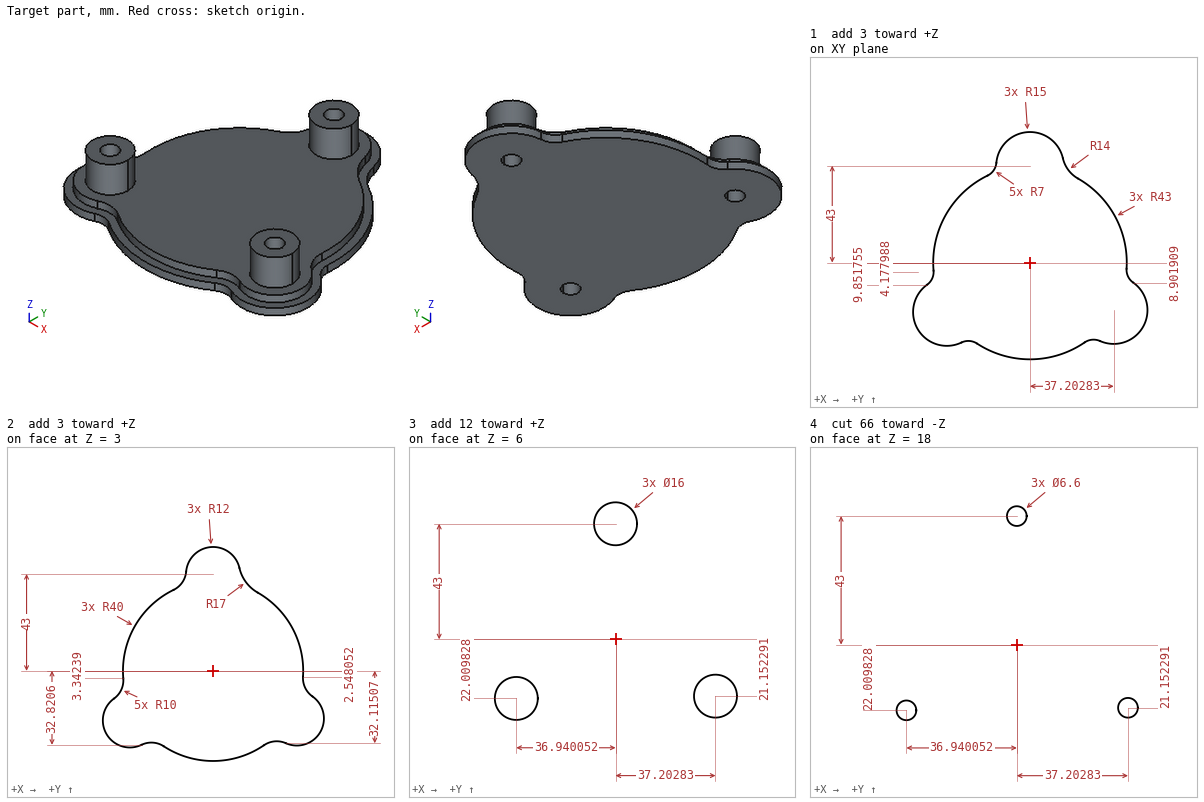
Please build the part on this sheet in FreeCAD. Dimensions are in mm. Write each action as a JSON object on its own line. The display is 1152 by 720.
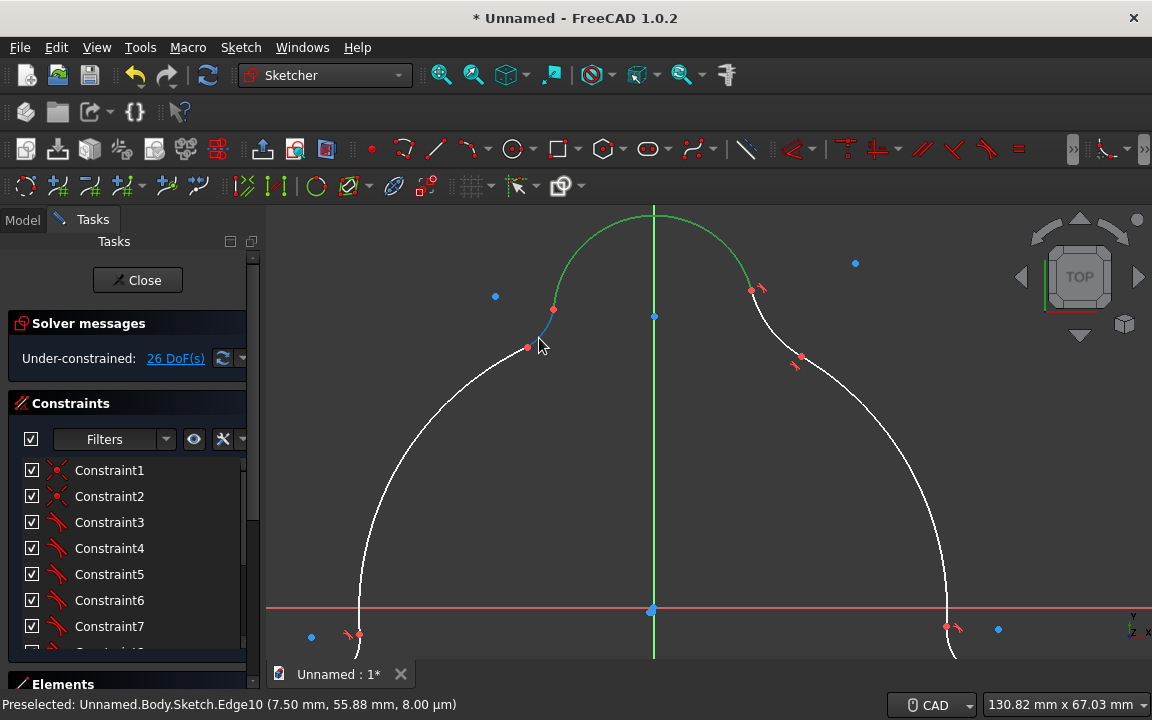
{"action": "left_click", "coordinate": [538, 338]}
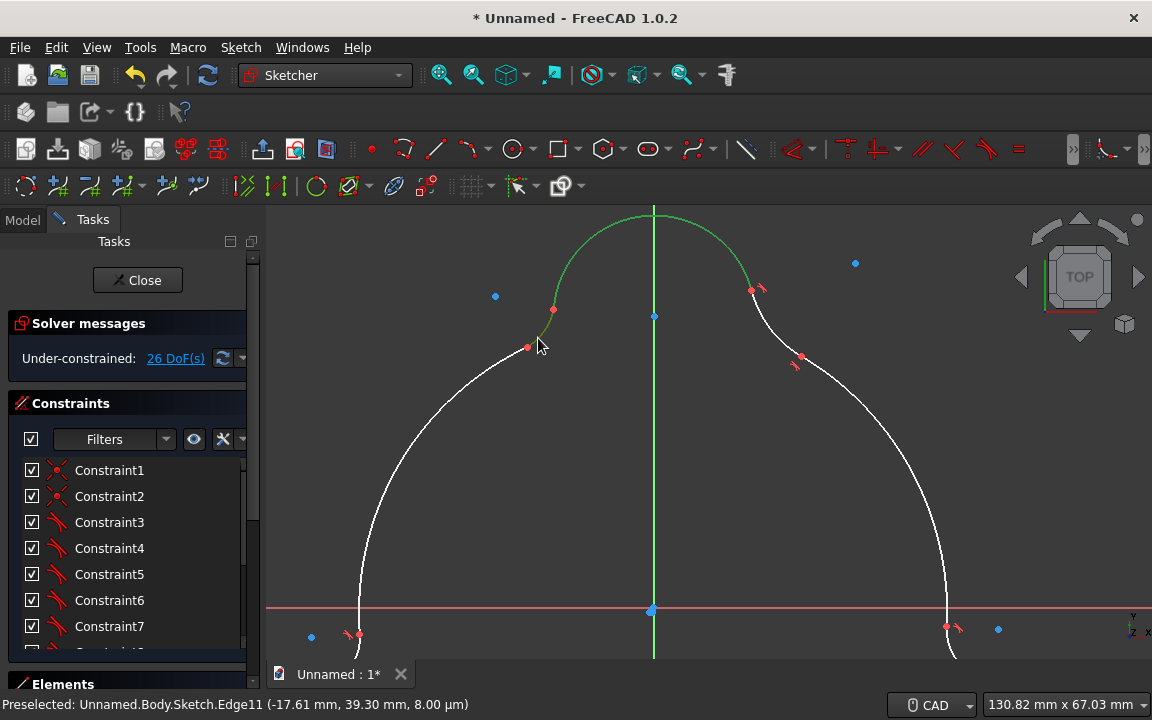
{"action": "left_click", "coordinate": [988, 150]}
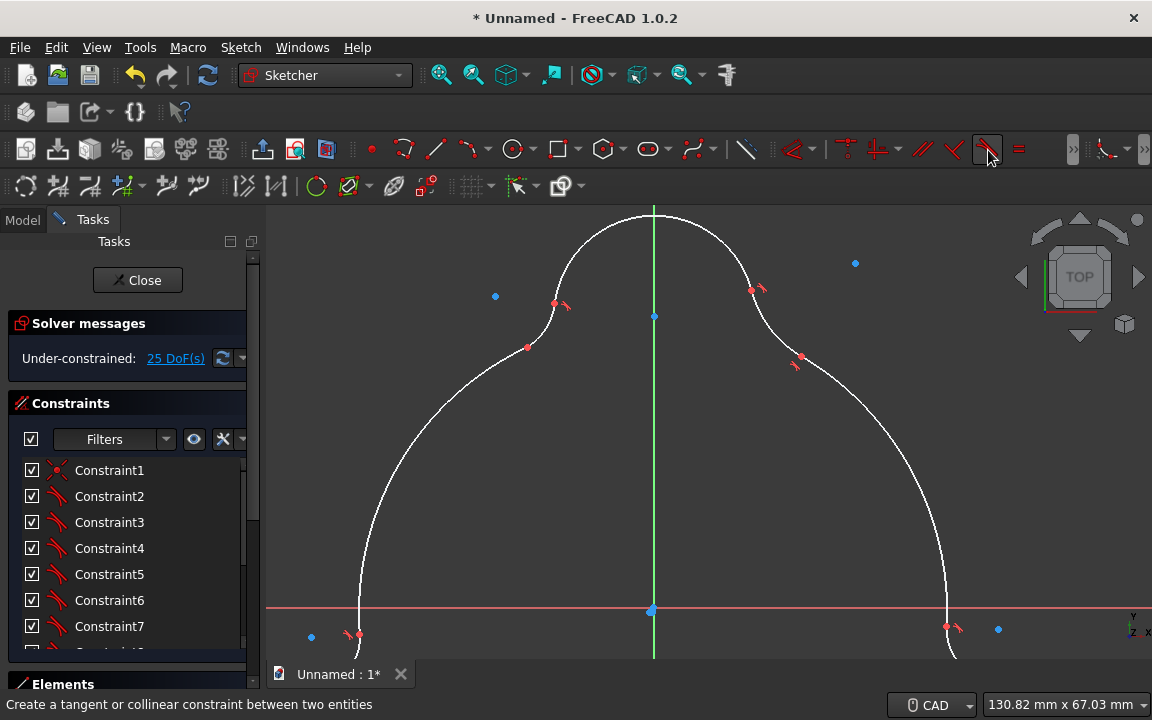
{"action": "left_click", "coordinate": [539, 337]}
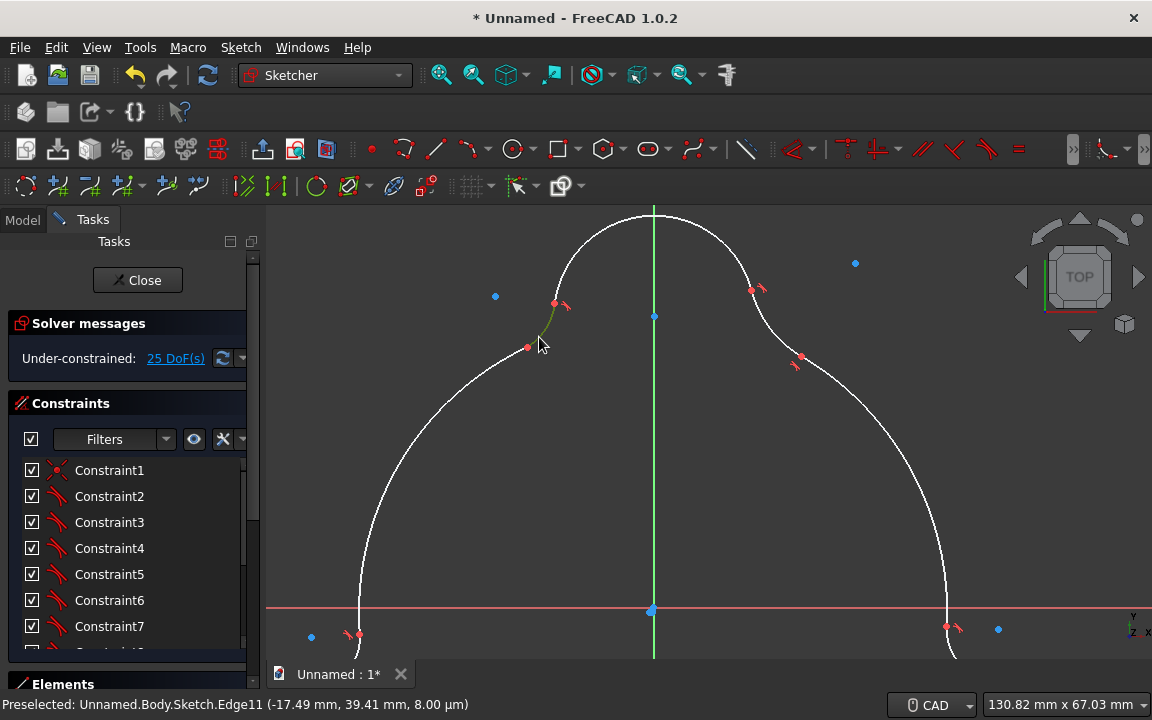
{"action": "left_click", "coordinate": [441, 408]}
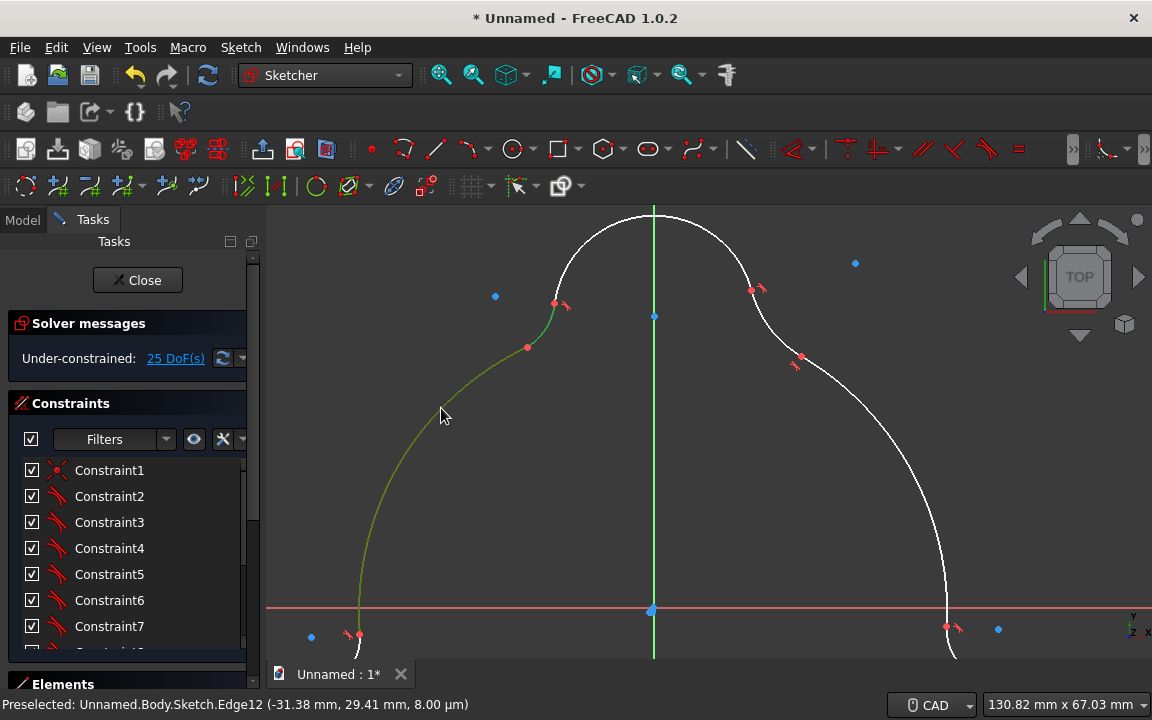
{"action": "left_click", "coordinate": [988, 150]}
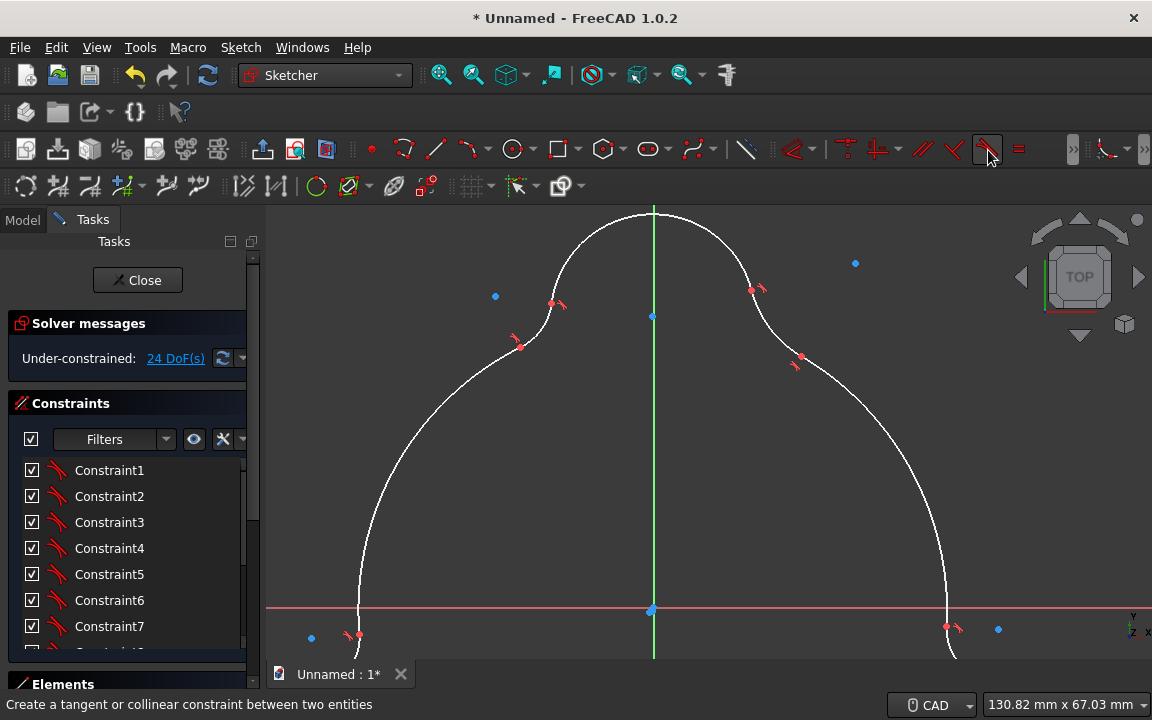
{"action": "scroll", "coordinate": [628, 330], "scroll_direction": "down", "scroll_amount": 4}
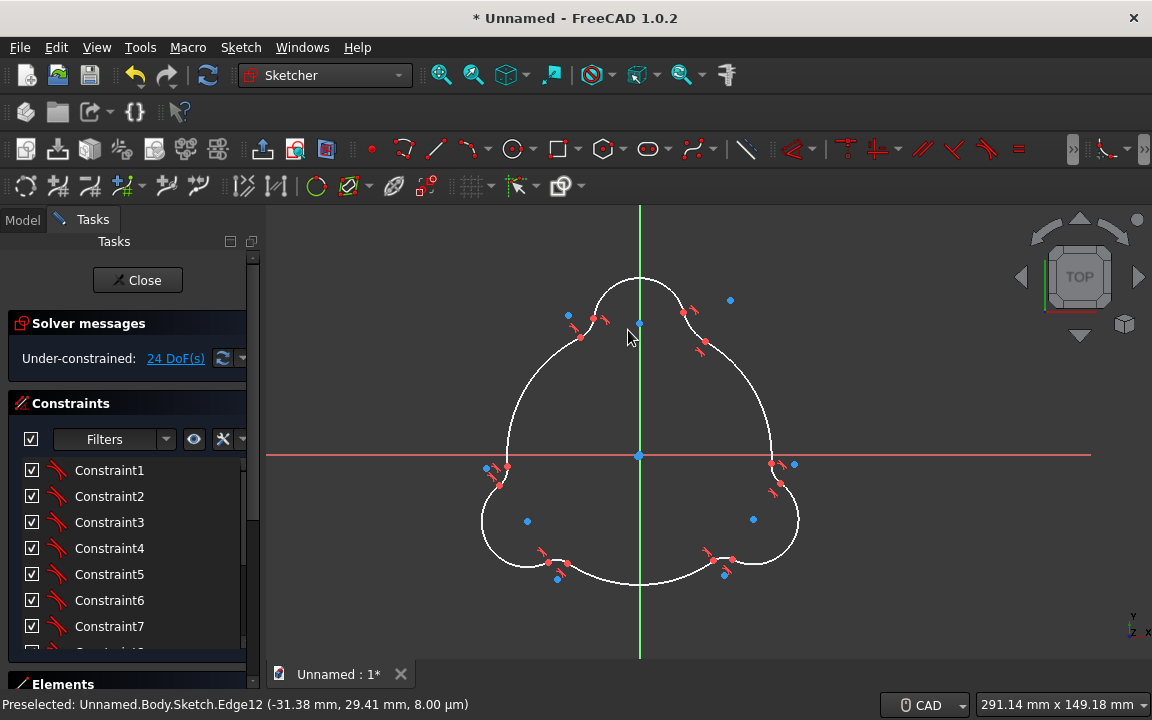
{"action": "left_click", "coordinate": [610, 582]}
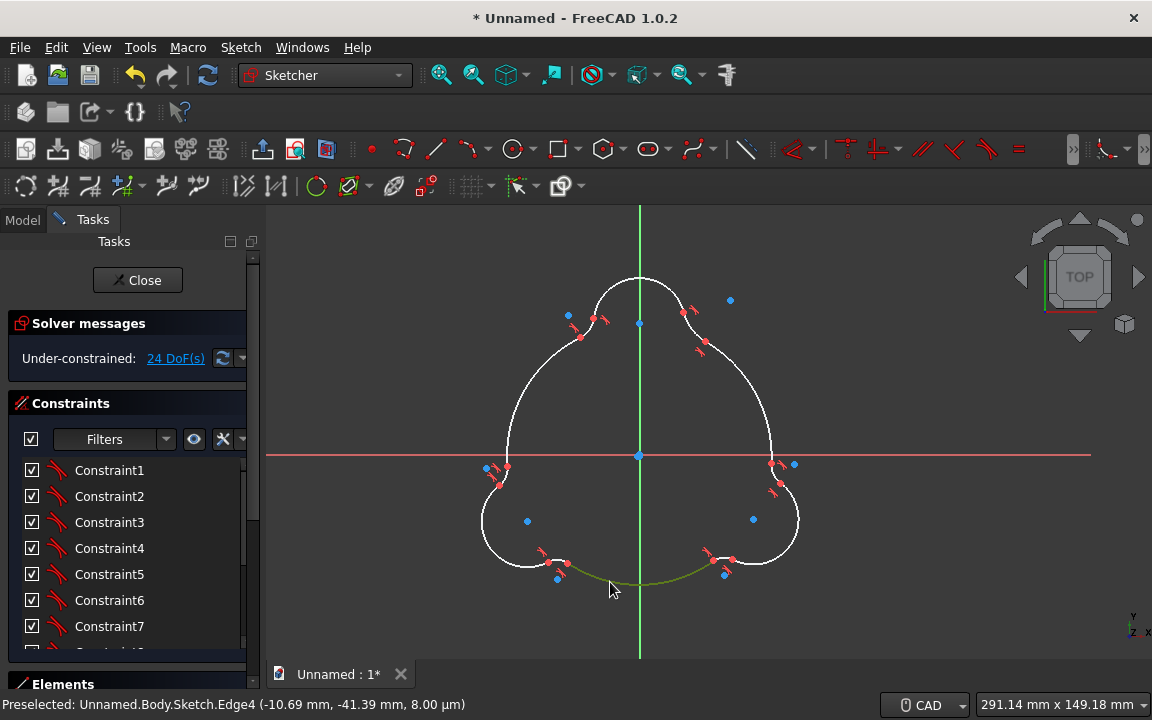
{"action": "left_click", "coordinate": [767, 420]}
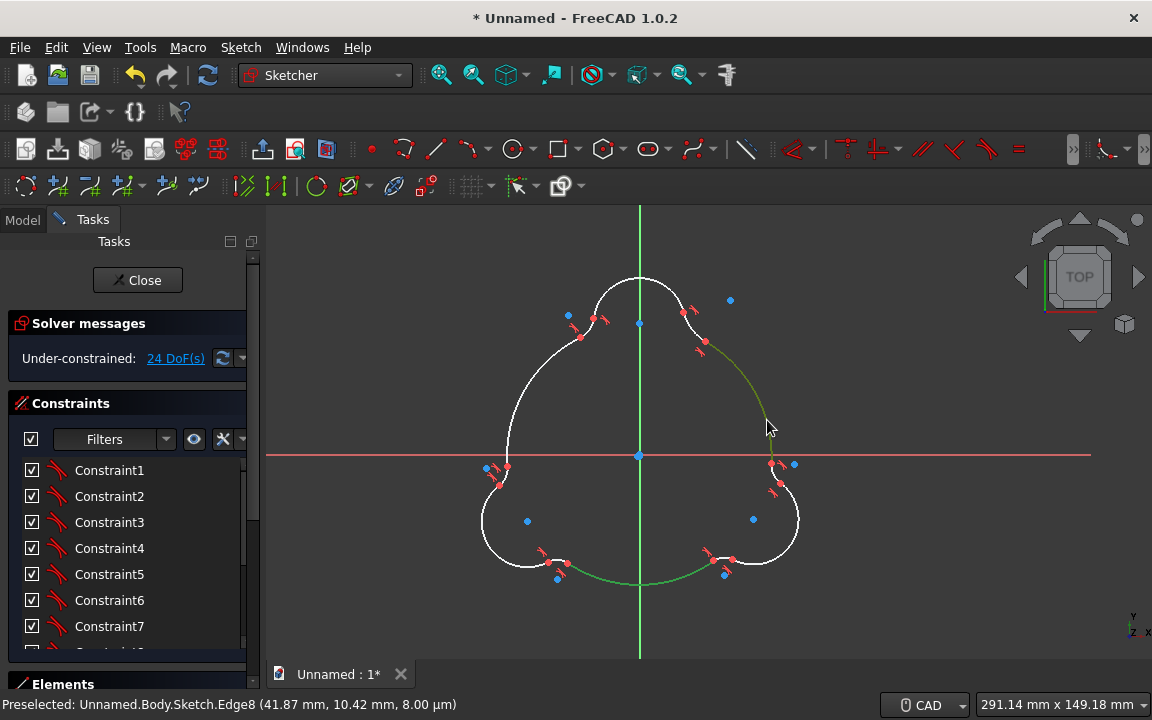
{"action": "left_click", "coordinate": [846, 150]}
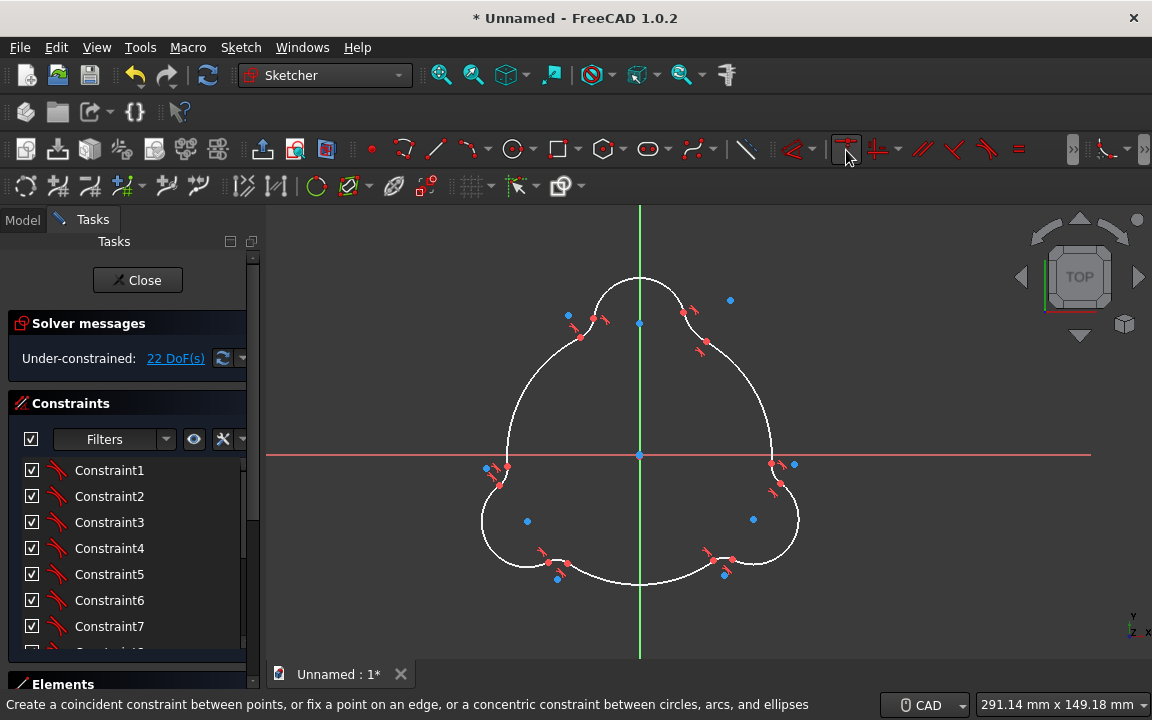
{"action": "left_click", "coordinate": [610, 582]}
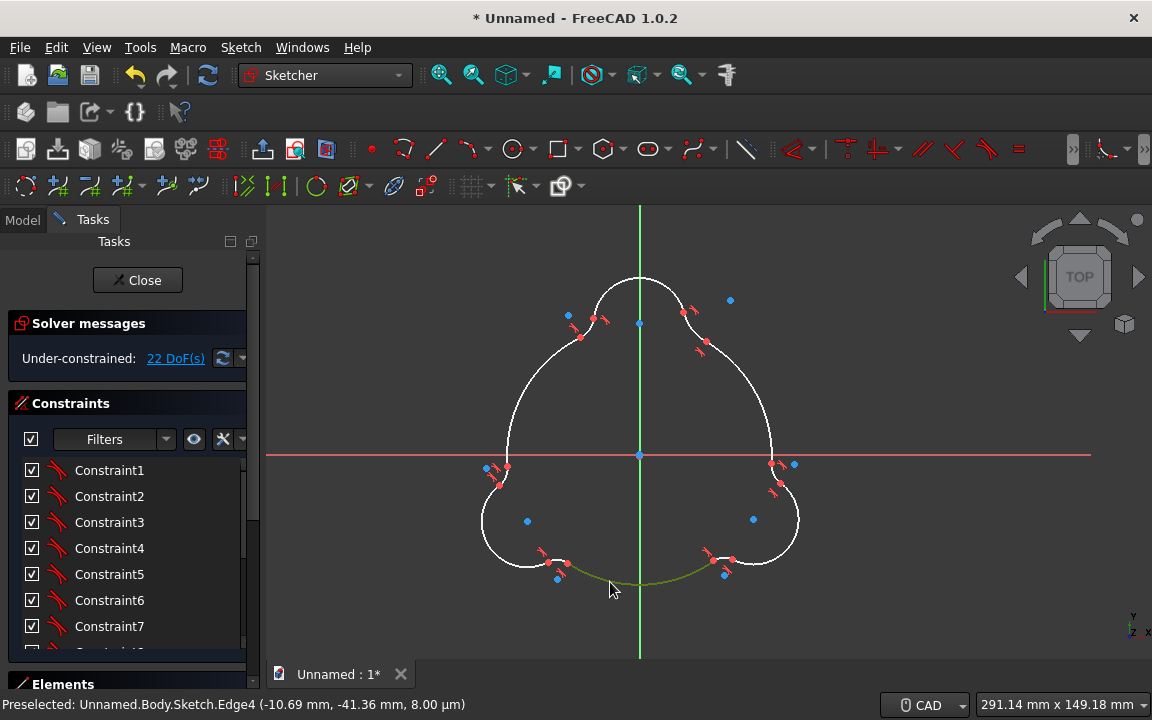
{"action": "left_click", "coordinate": [543, 366]}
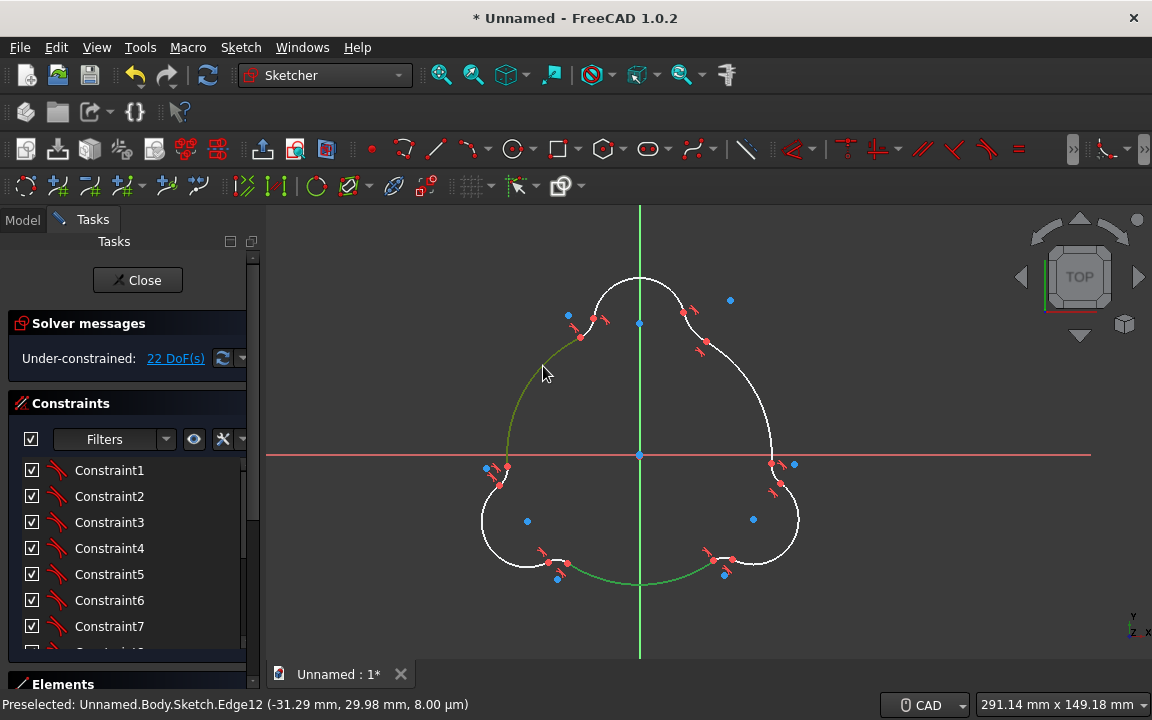
{"action": "left_click", "coordinate": [846, 150]}